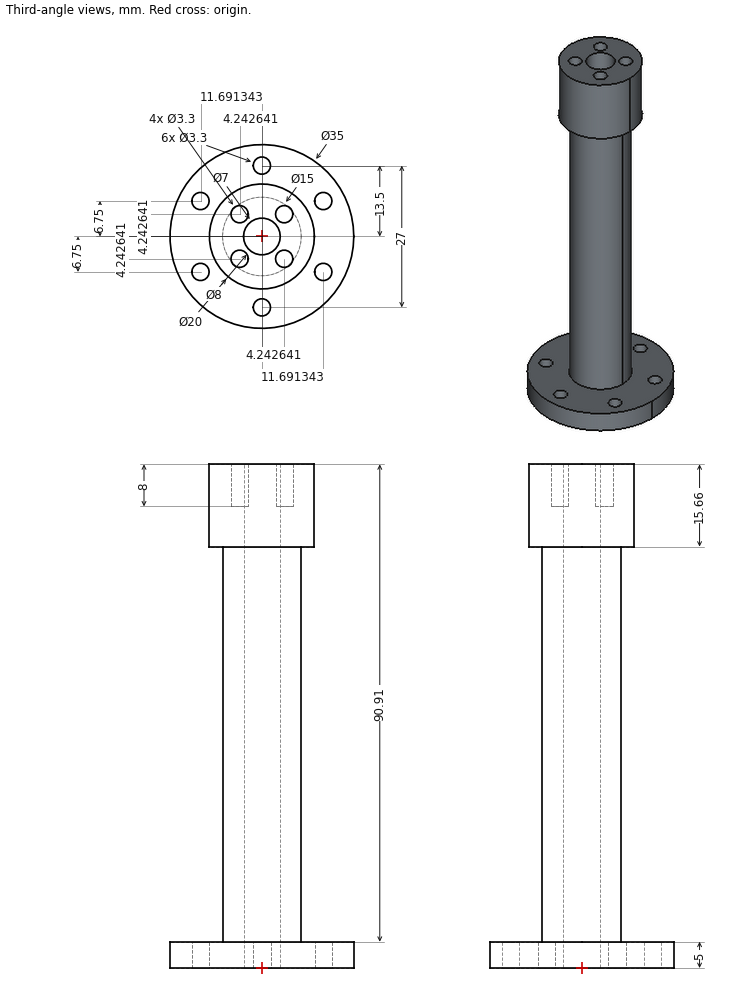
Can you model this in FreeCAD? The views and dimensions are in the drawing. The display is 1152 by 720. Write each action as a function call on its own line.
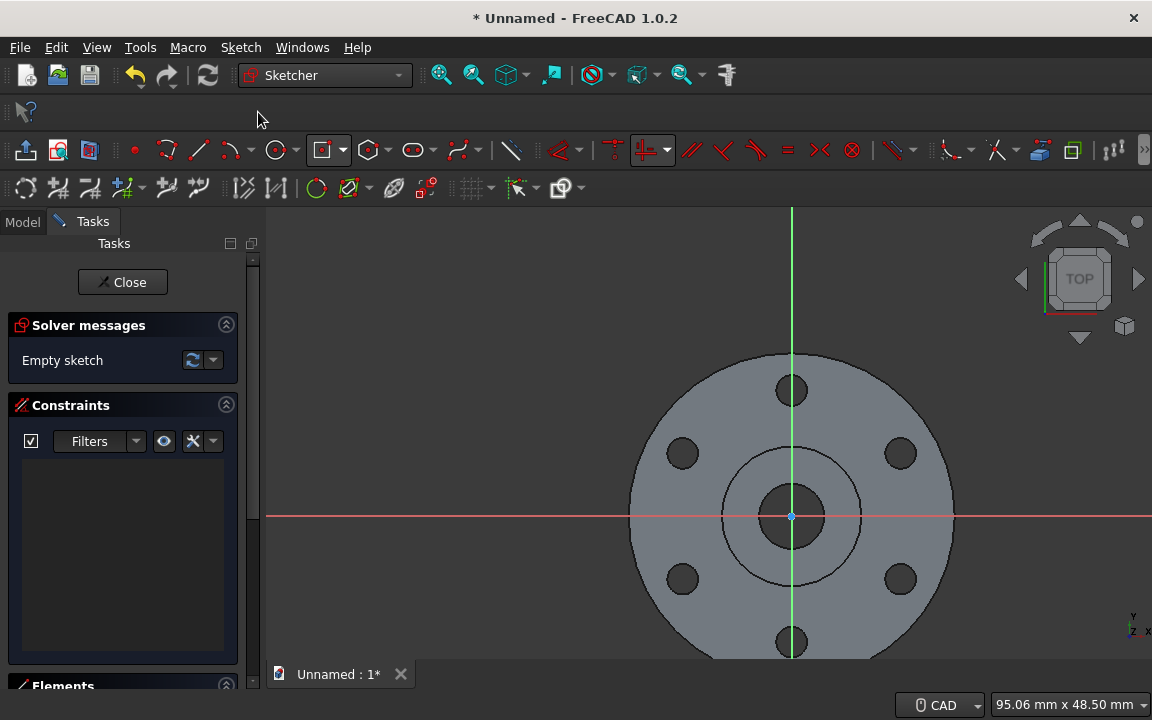
scroll(987, 631, up, 2)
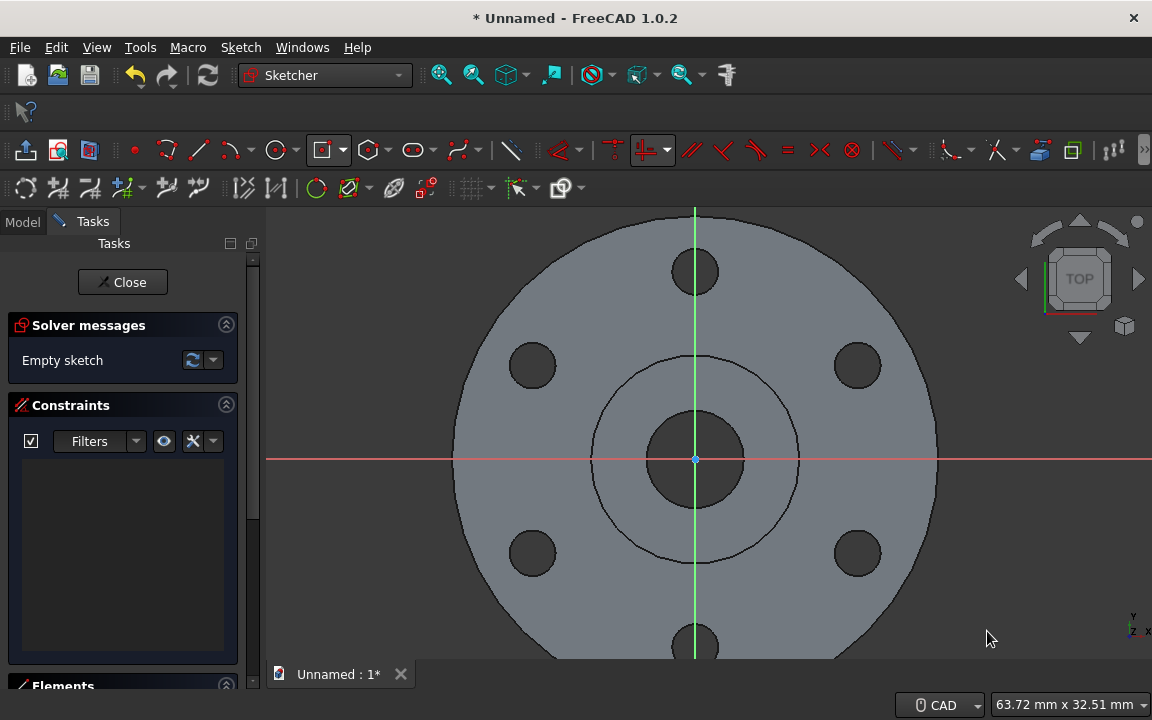
key(g)
key(c)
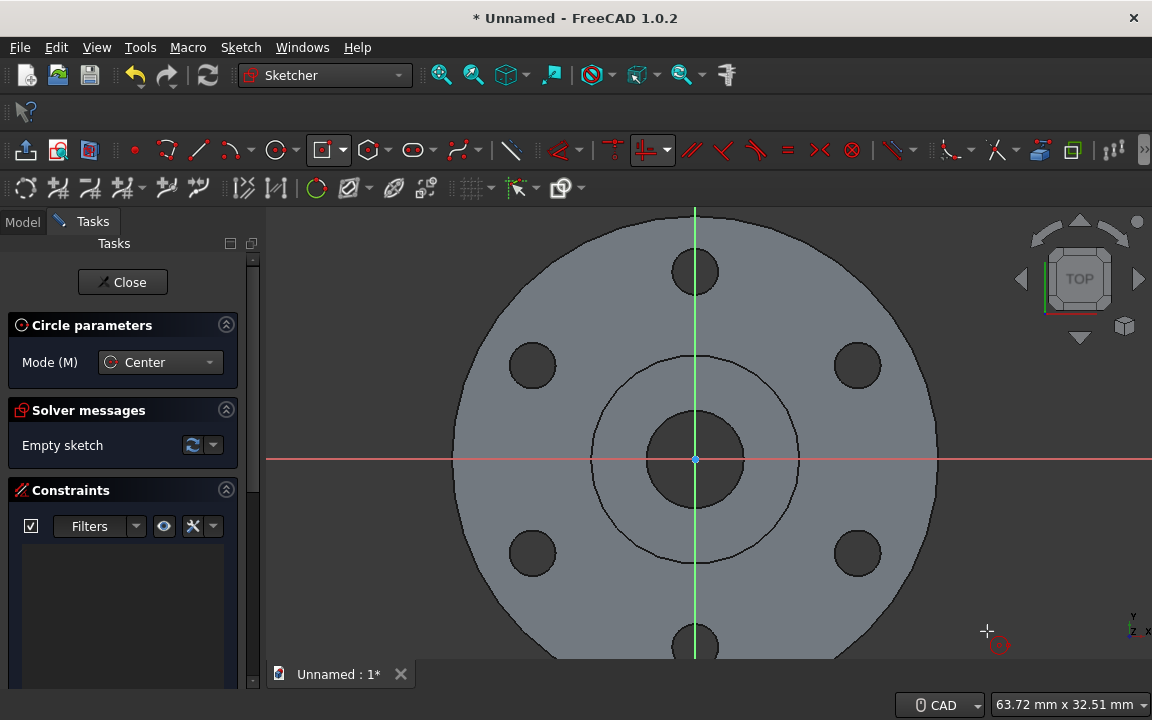
click(695, 459)
click(794, 361)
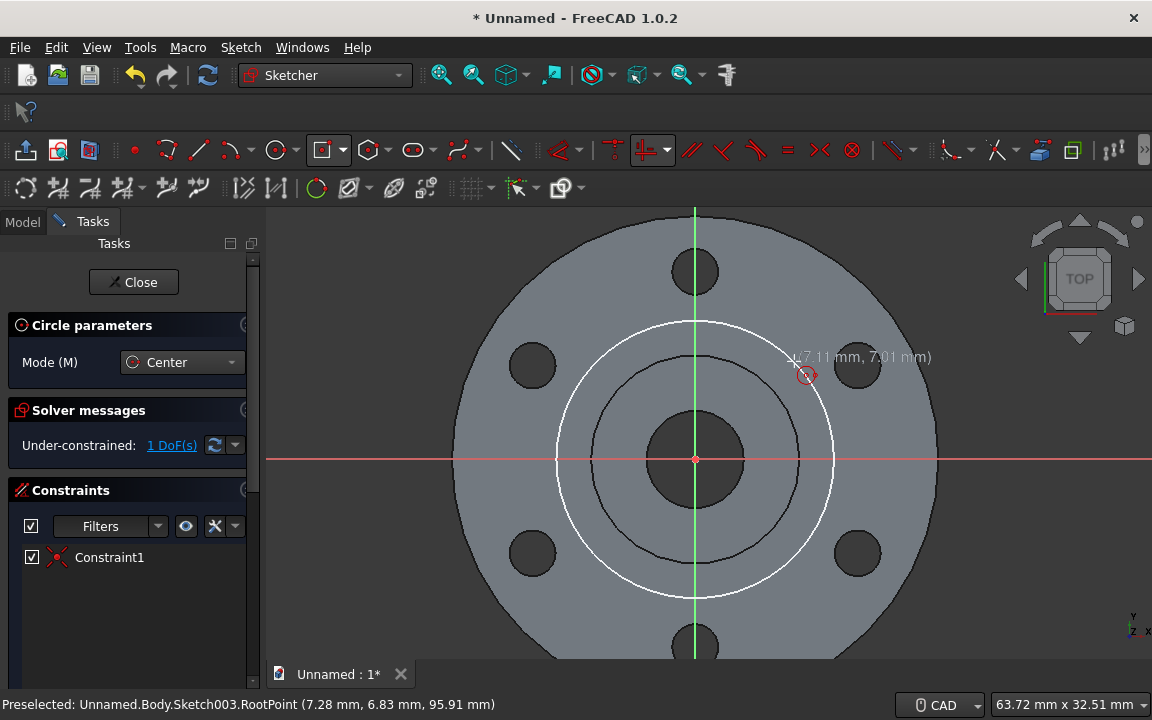
click(695, 459)
click(735, 420)
key(Escape)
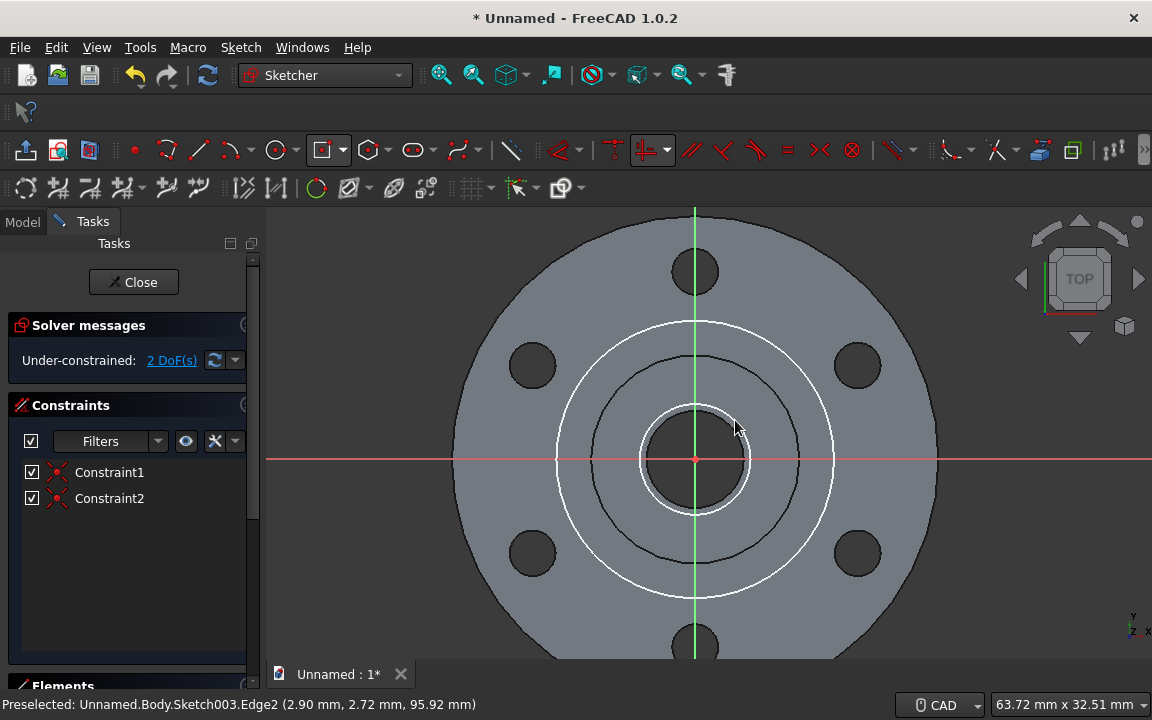
key(d)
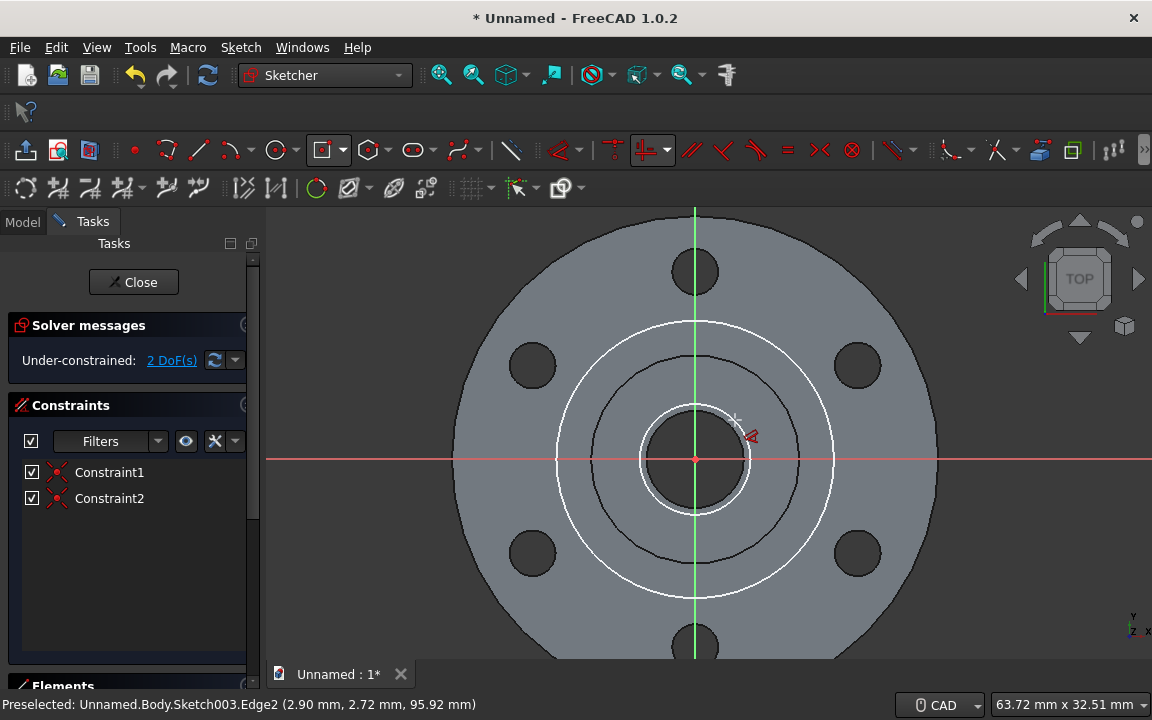
click(793, 361)
click(816, 338)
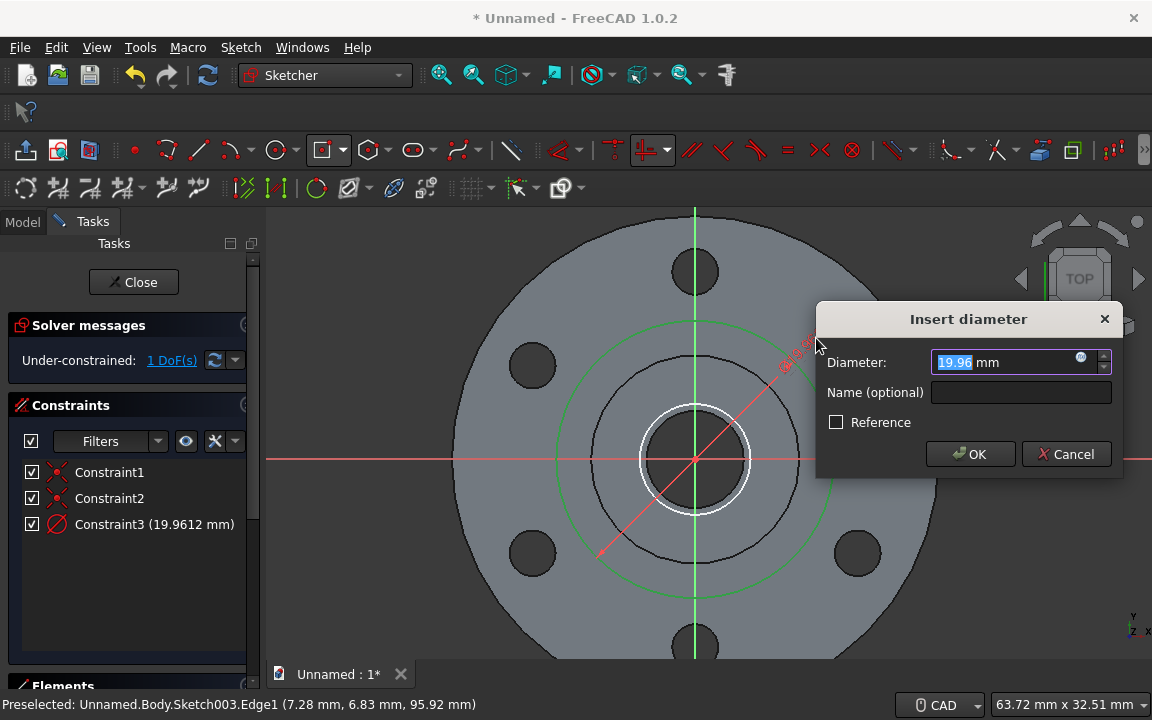
text(20)
key(Return)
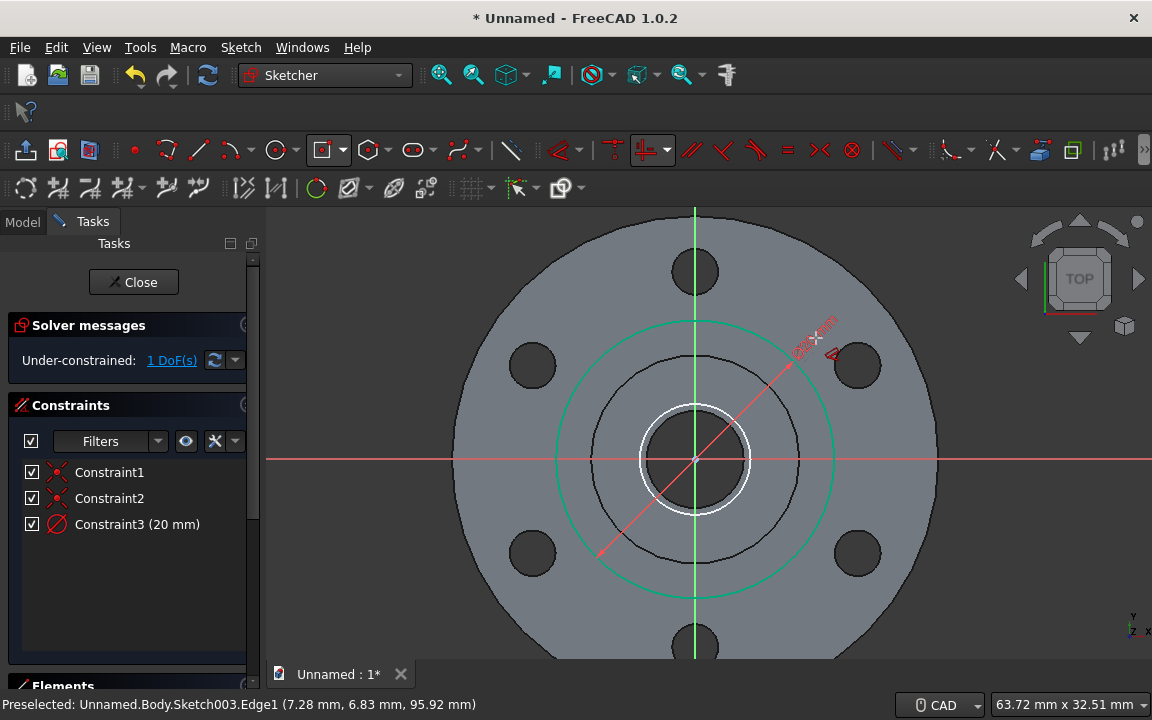
click(734, 420)
click(756, 397)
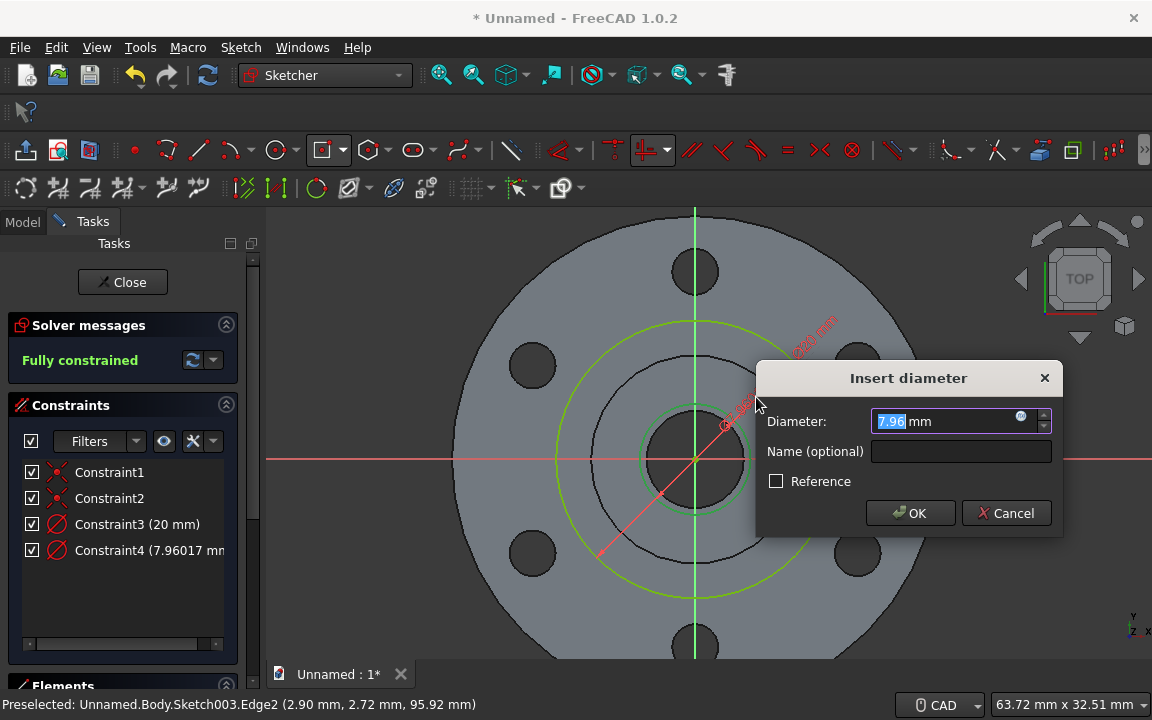
text(8)
key(Return)
key(Escape)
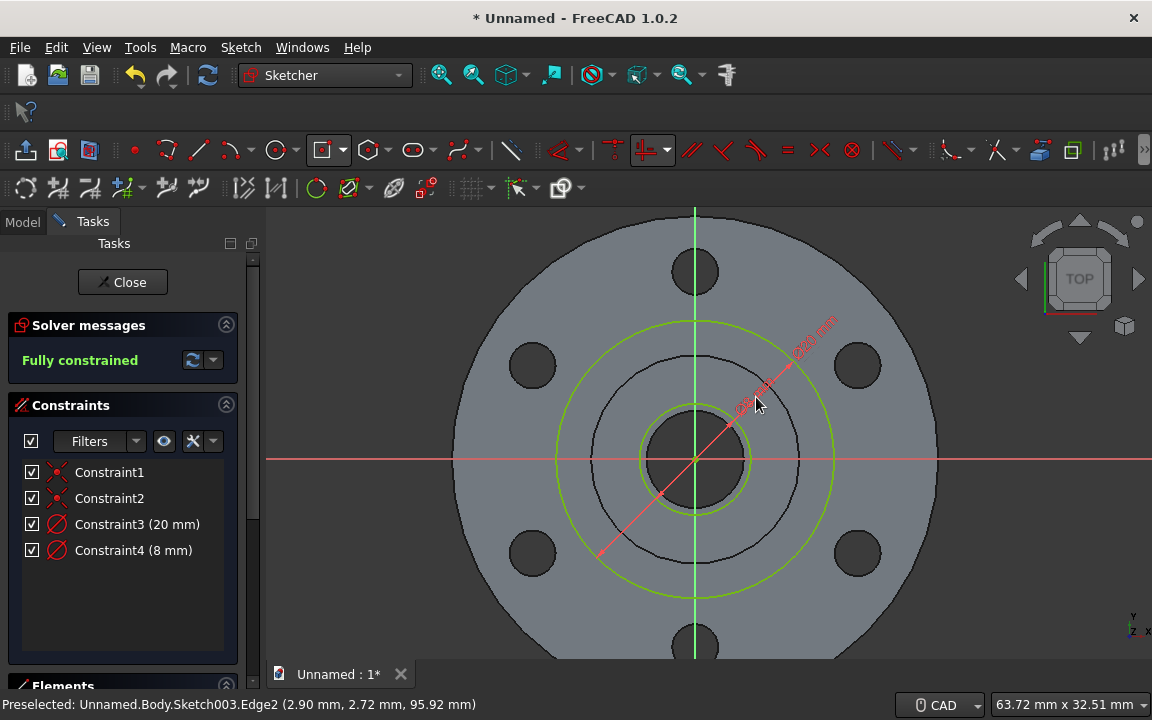
click(123, 282)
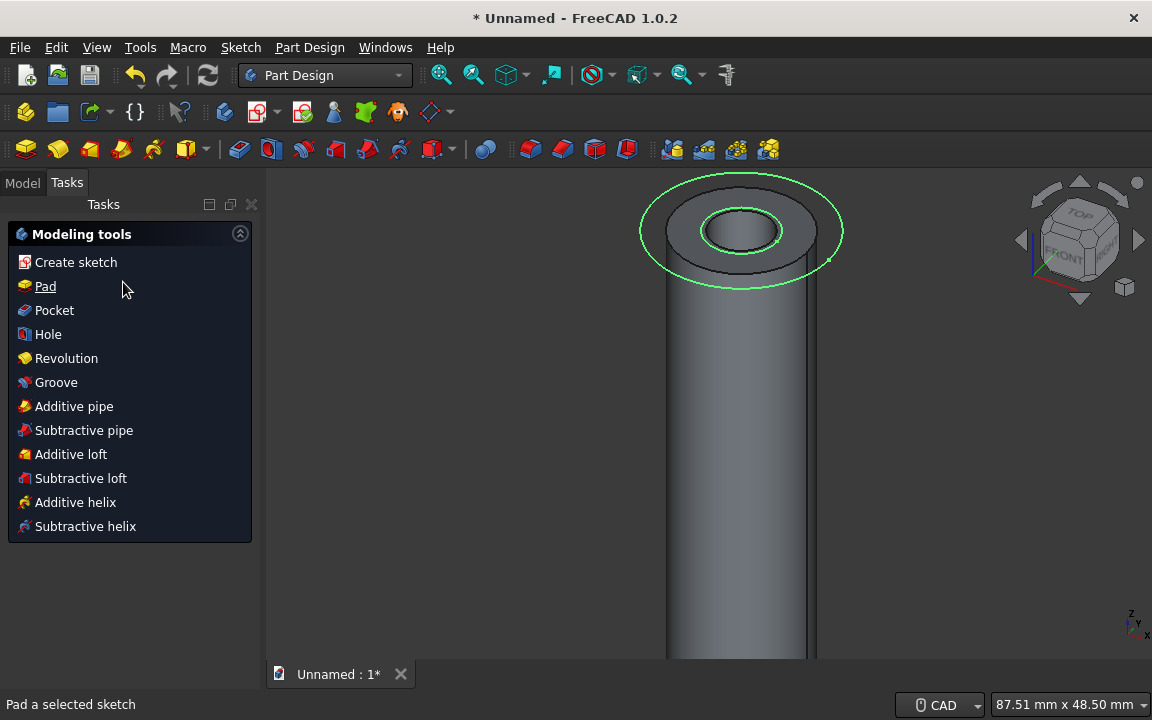
click(26, 150)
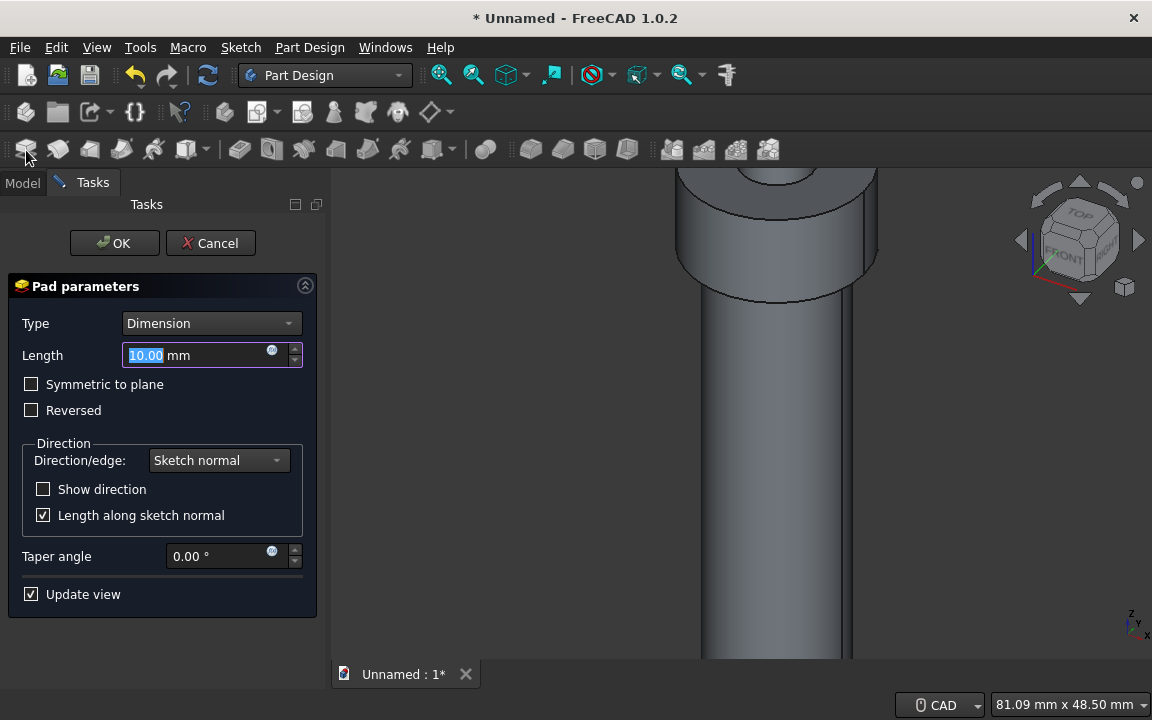
text(15.66)
key(Tab)